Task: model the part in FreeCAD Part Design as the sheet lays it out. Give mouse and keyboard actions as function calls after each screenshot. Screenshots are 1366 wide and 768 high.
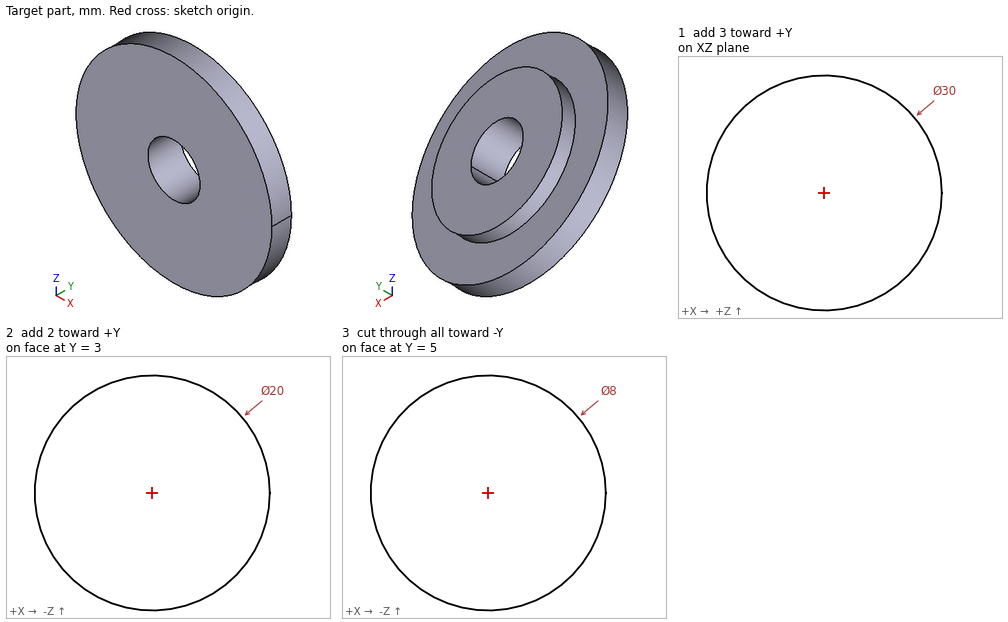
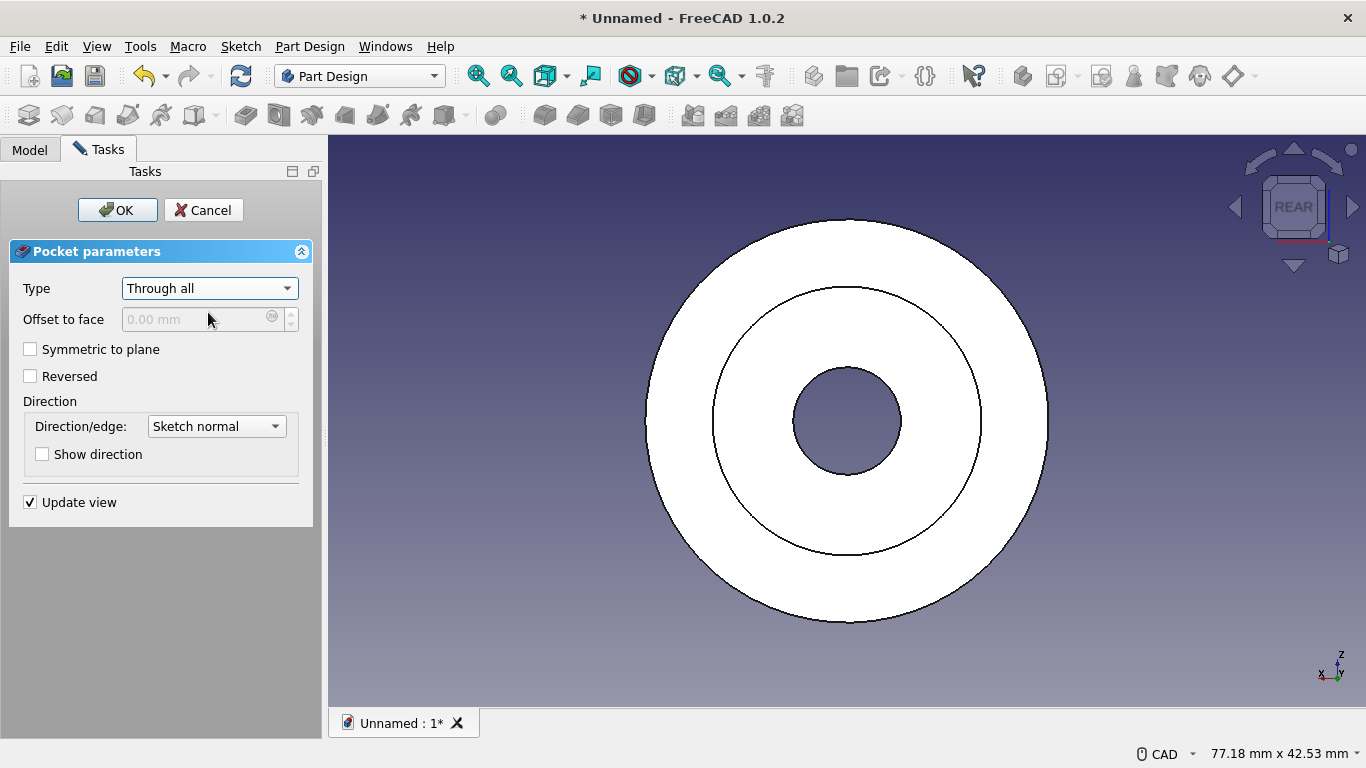
click(118, 210)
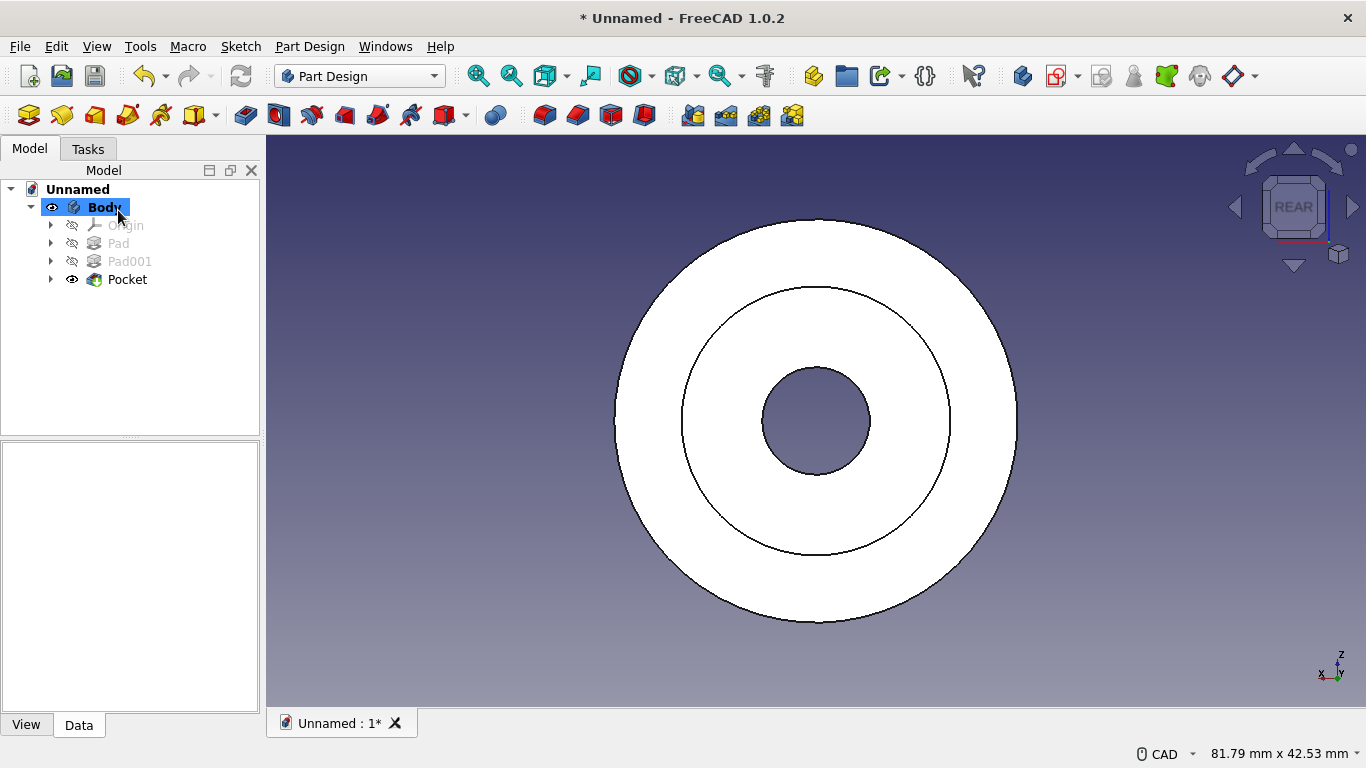
key(0)